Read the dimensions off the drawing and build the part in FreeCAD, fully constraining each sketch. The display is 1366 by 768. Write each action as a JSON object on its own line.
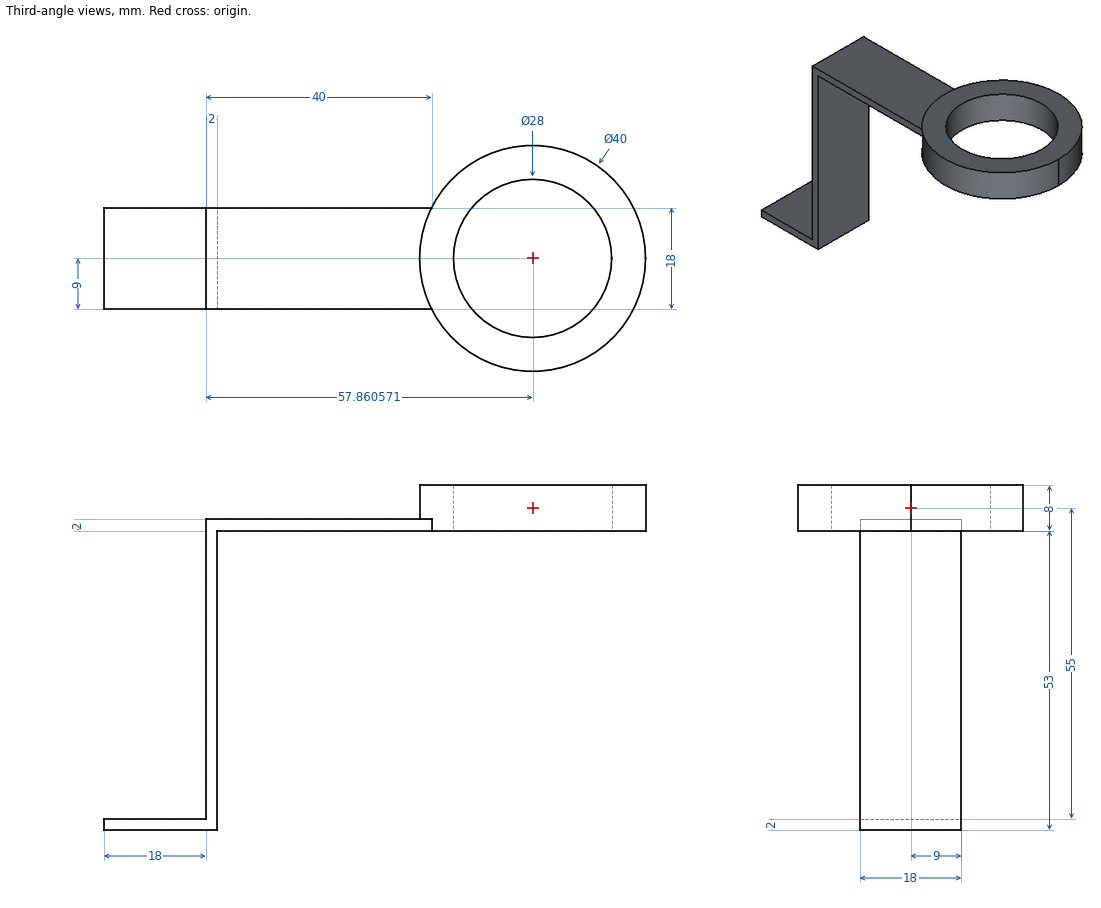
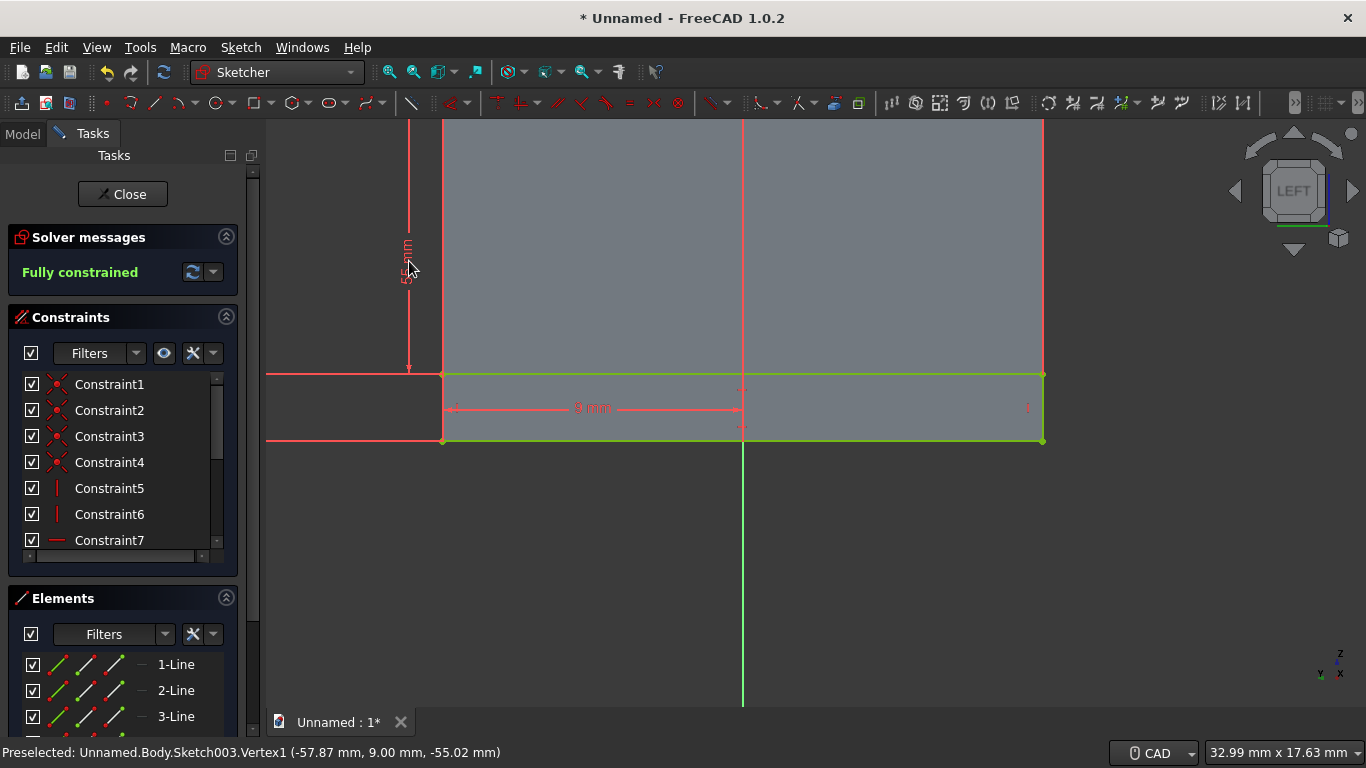
{"action": "left_click", "coordinate": [123, 194]}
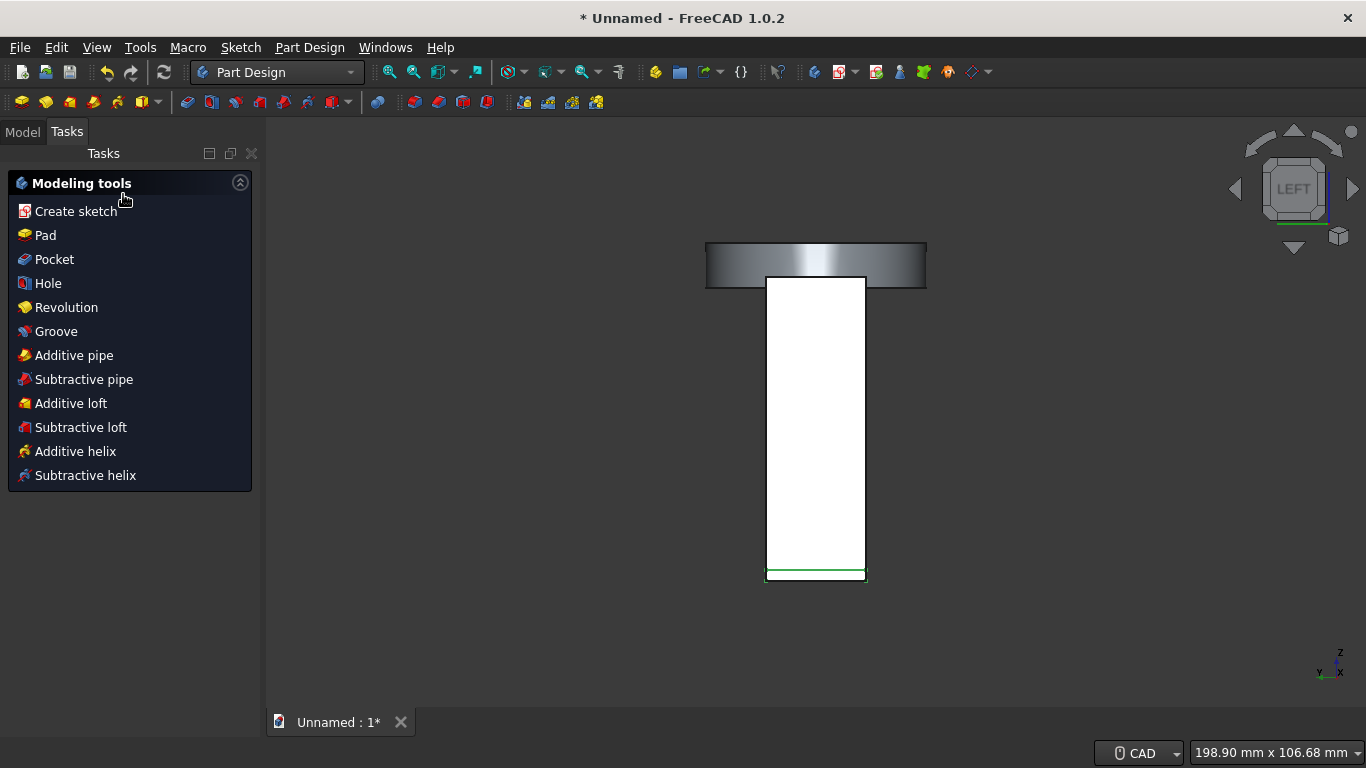
{"action": "left_click", "coordinate": [22, 102]}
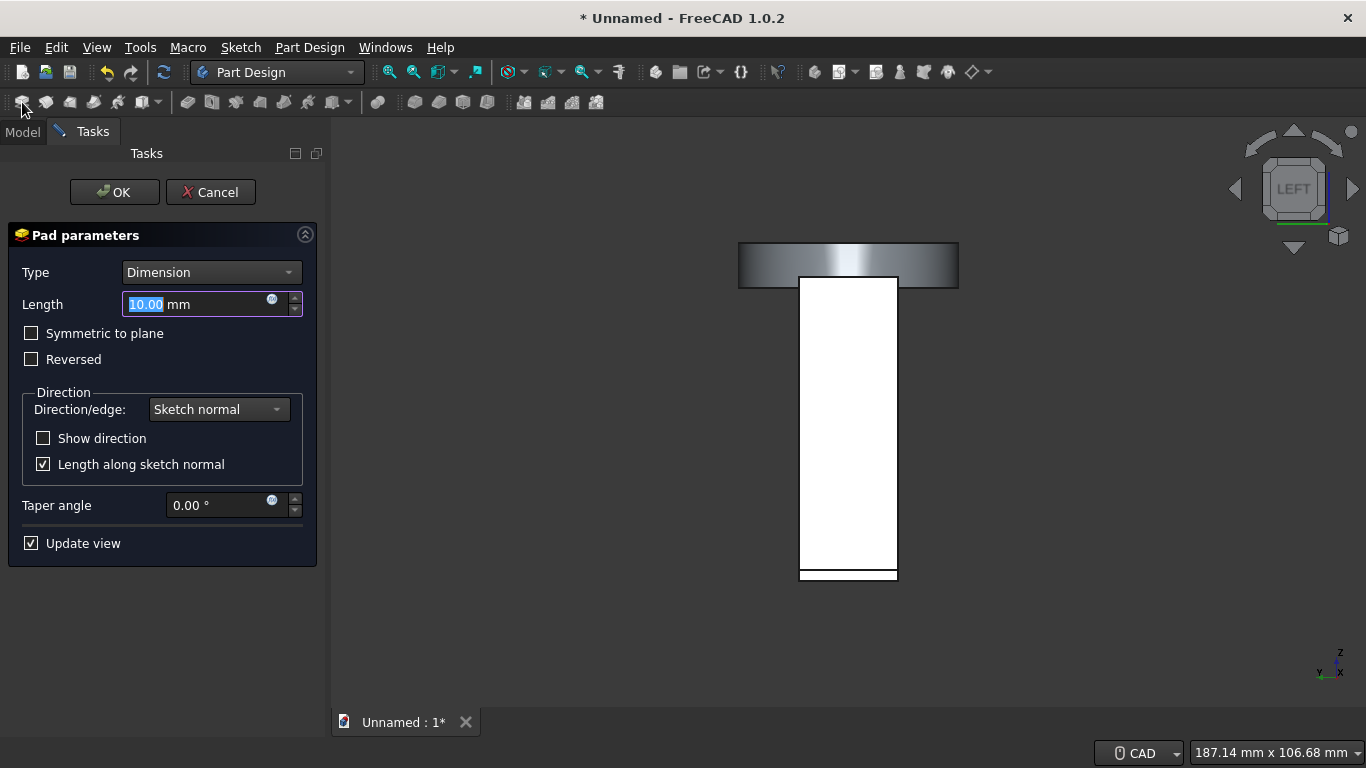
{"action": "type", "text": "18"}
{"action": "key", "text": "Tab"}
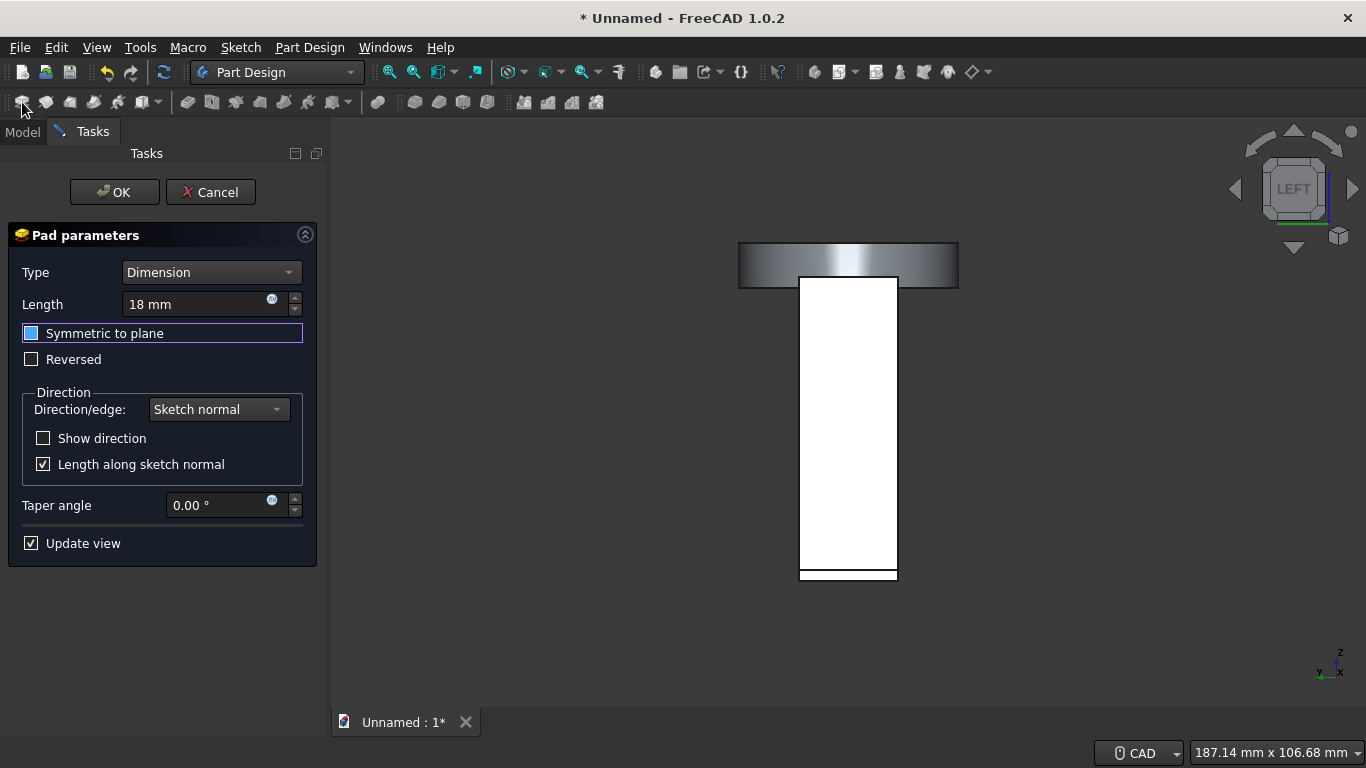
{"action": "left_click", "coordinate": [115, 192]}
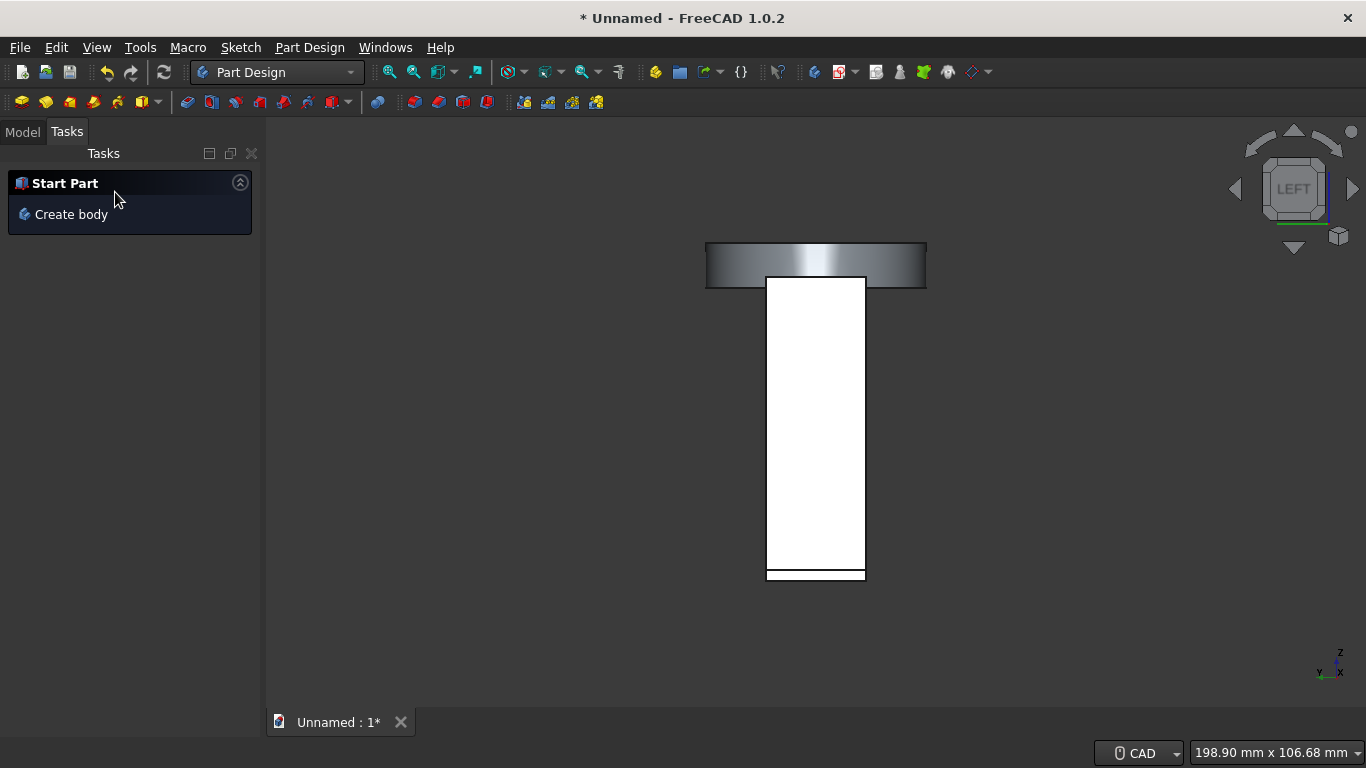
{"action": "key", "text": "0"}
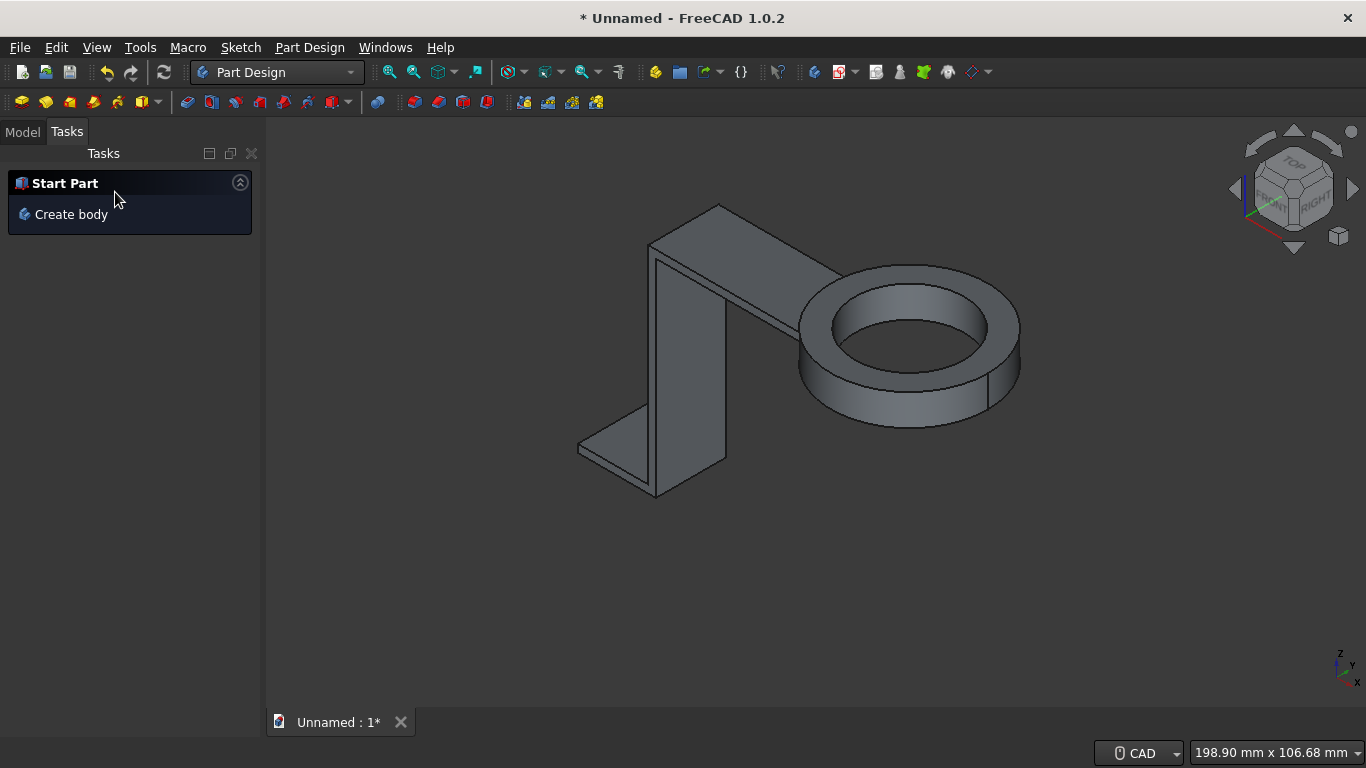
{"action": "left_click", "coordinate": [390, 72]}